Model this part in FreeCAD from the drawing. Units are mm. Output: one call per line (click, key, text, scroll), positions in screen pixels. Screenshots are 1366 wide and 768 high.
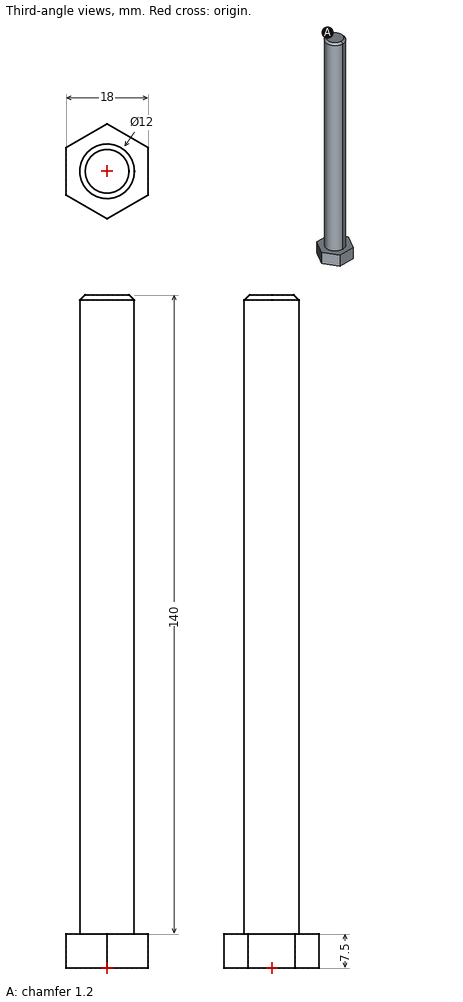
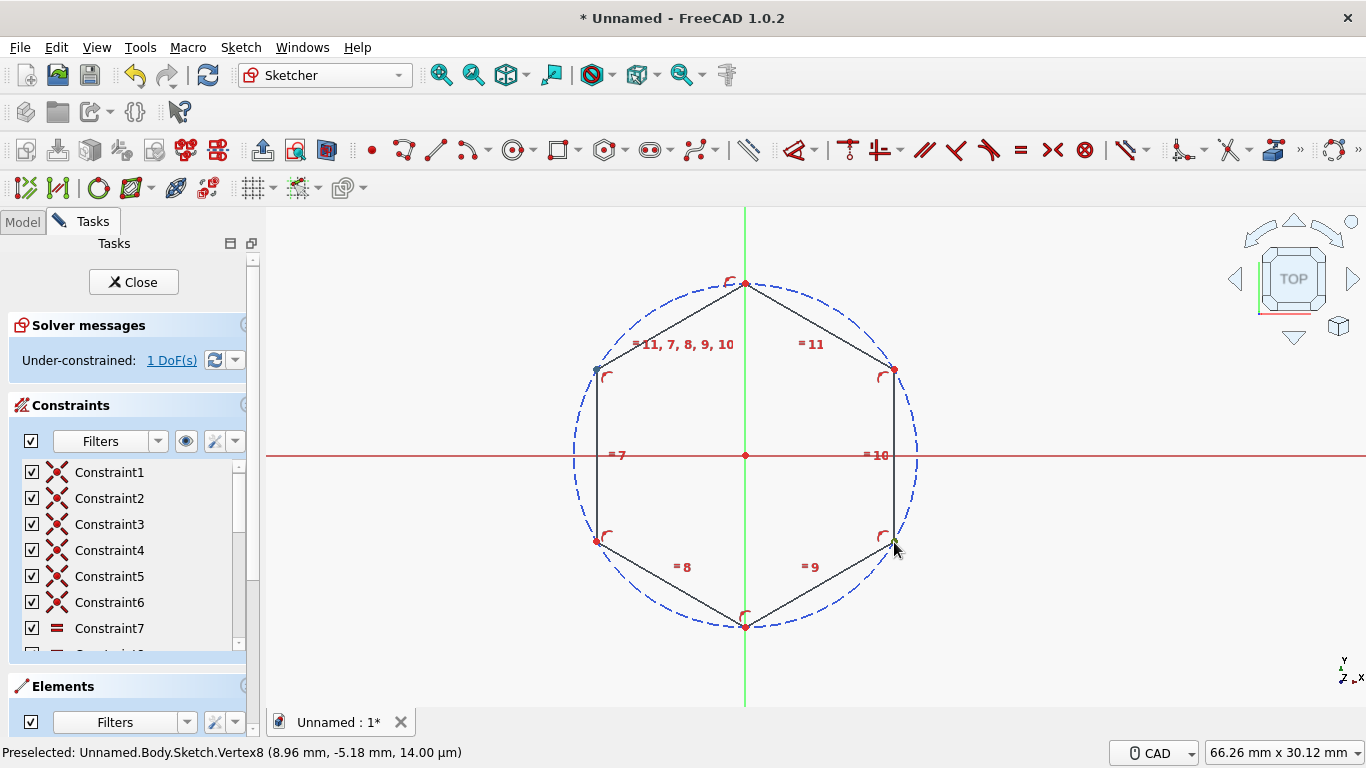
key(l)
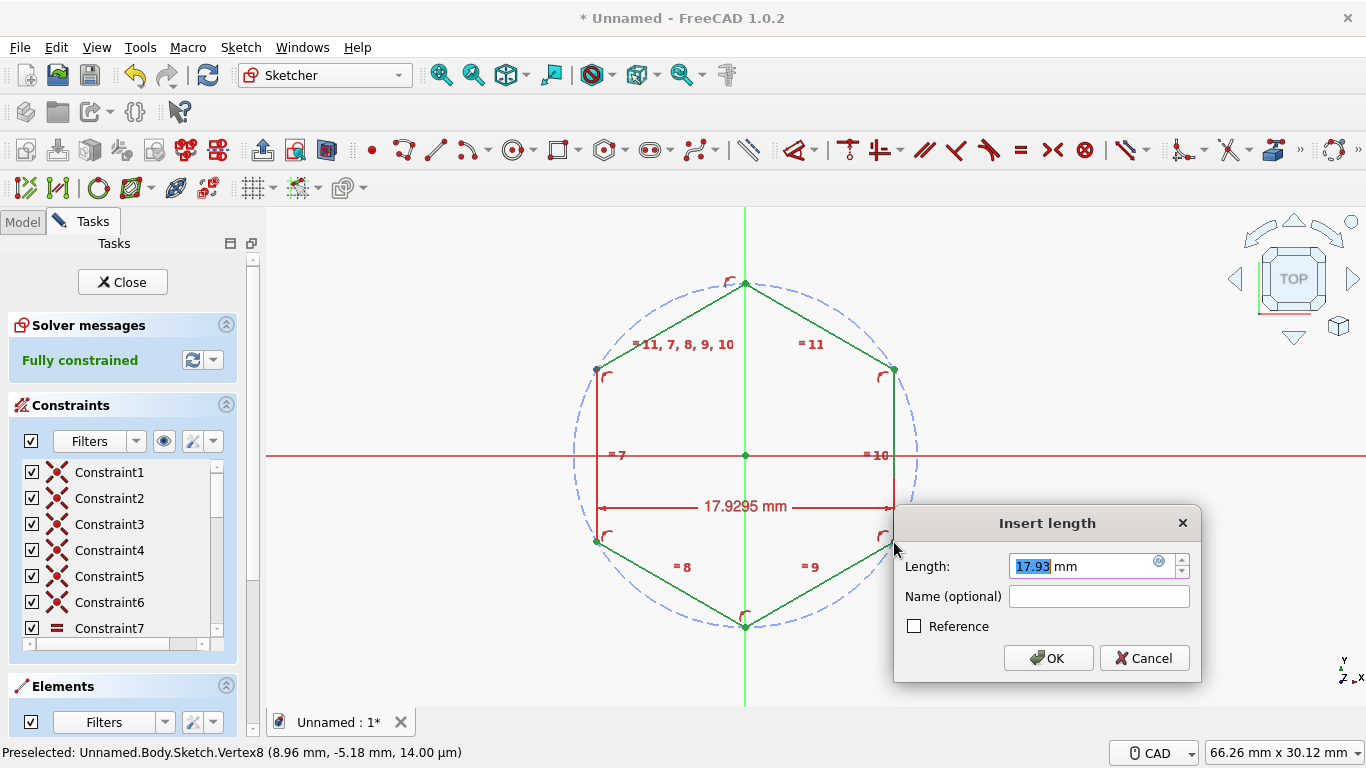
text(18)
key(Return)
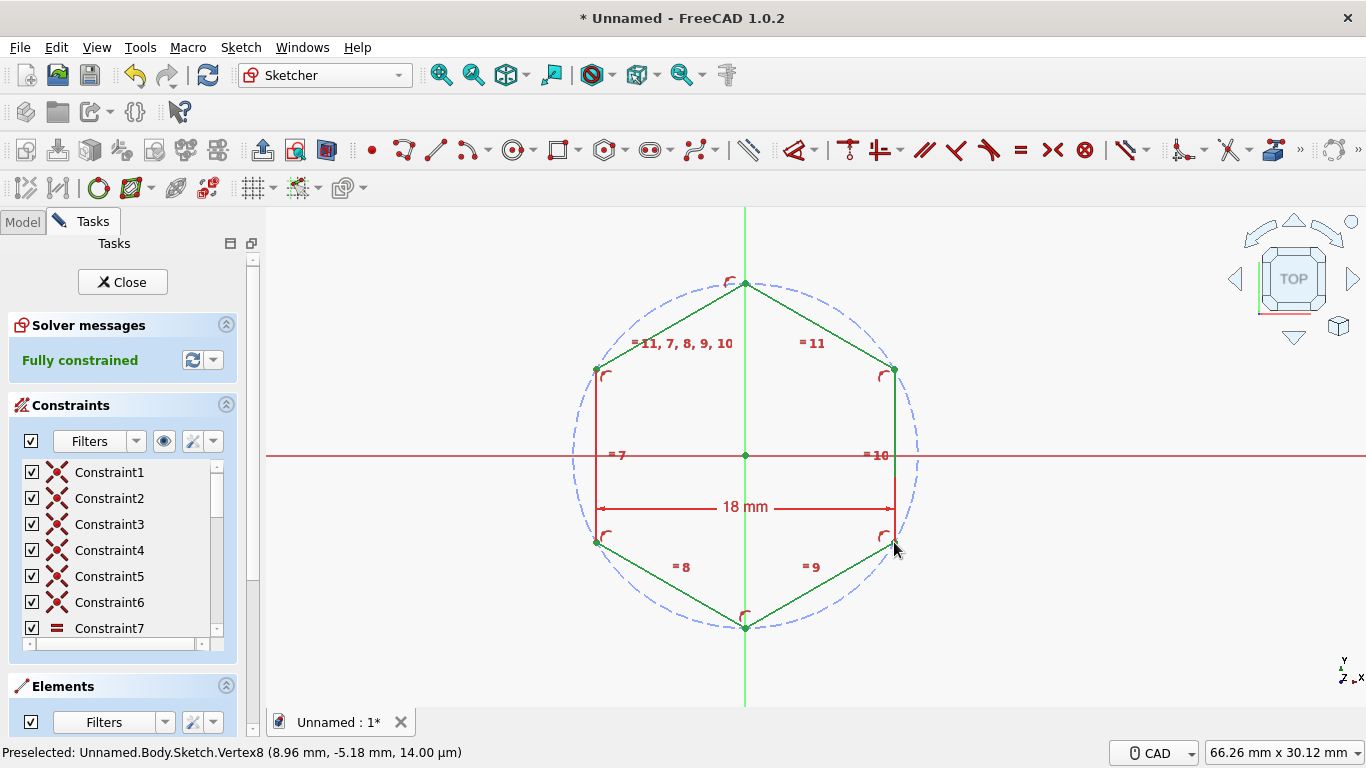
click(123, 282)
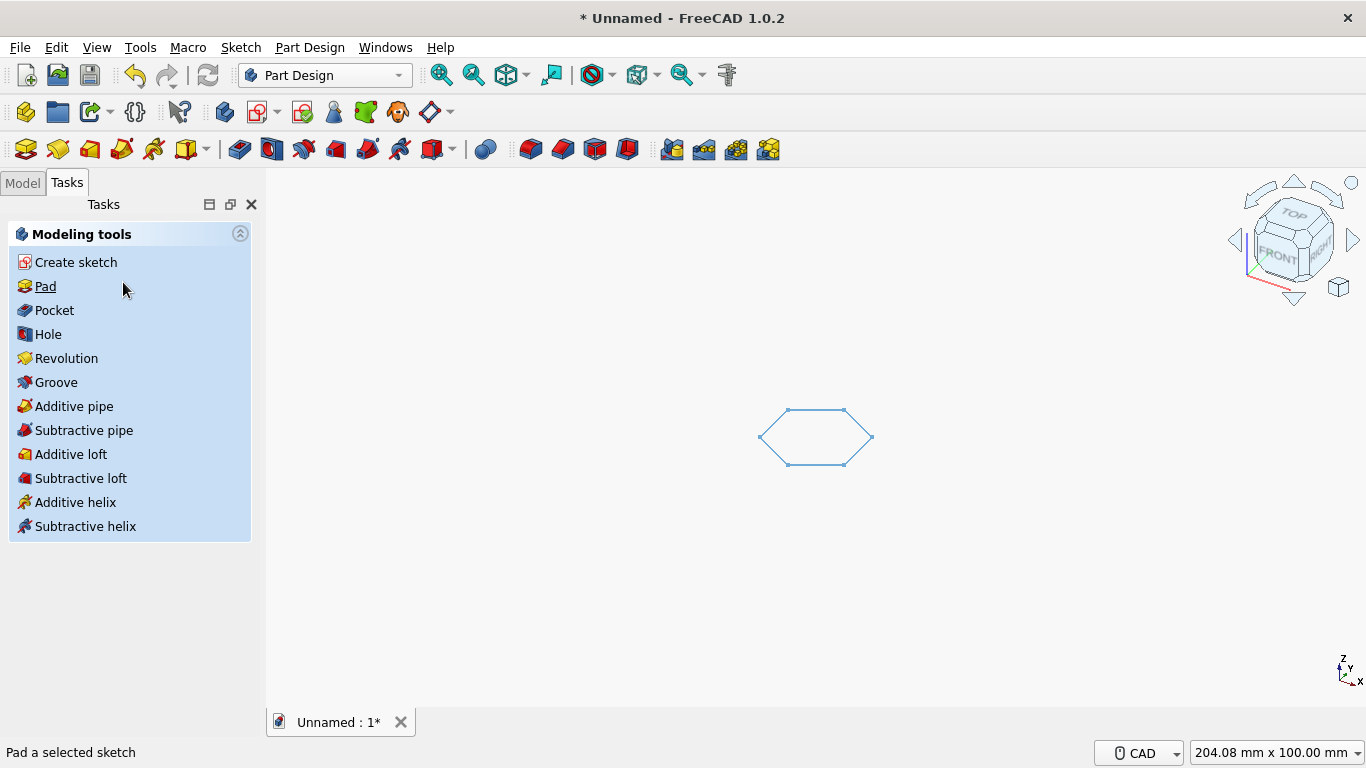
click(26, 150)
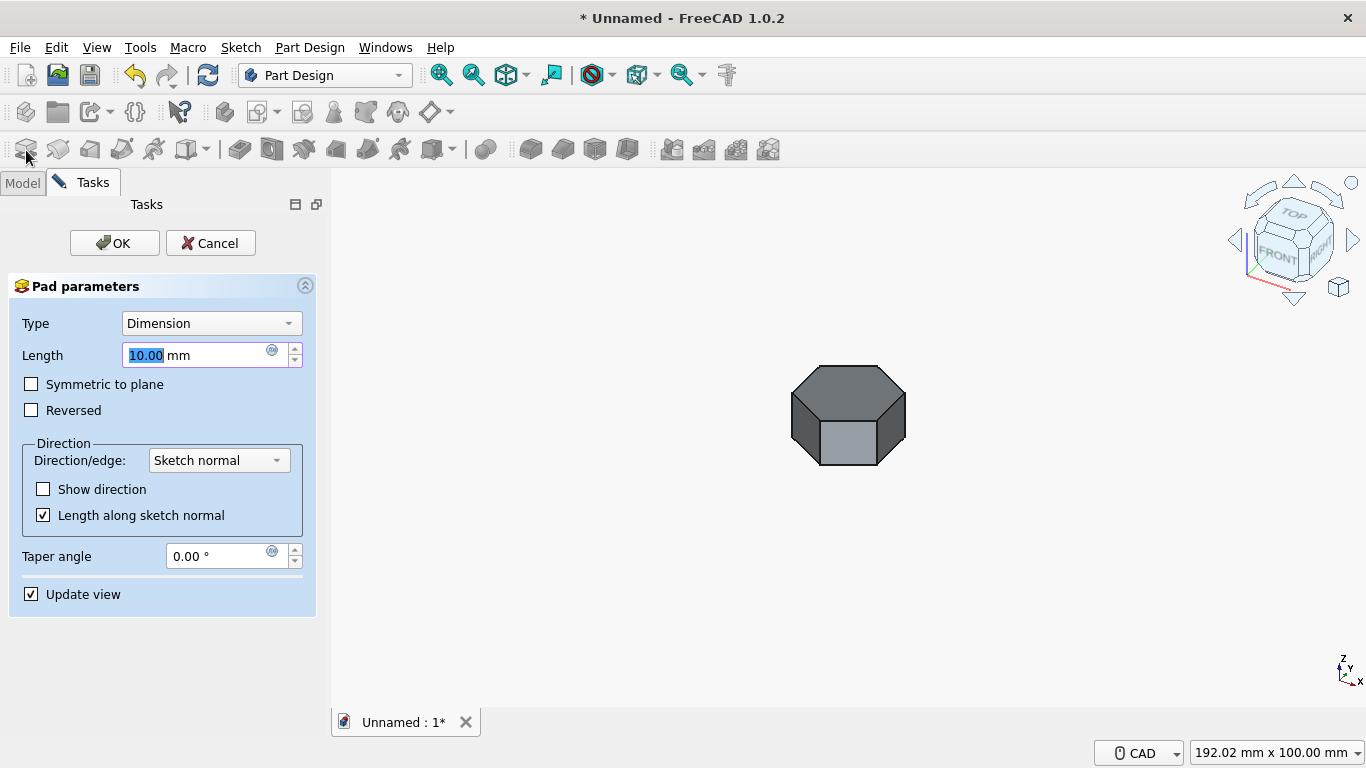
text(7.5)
key(Tab)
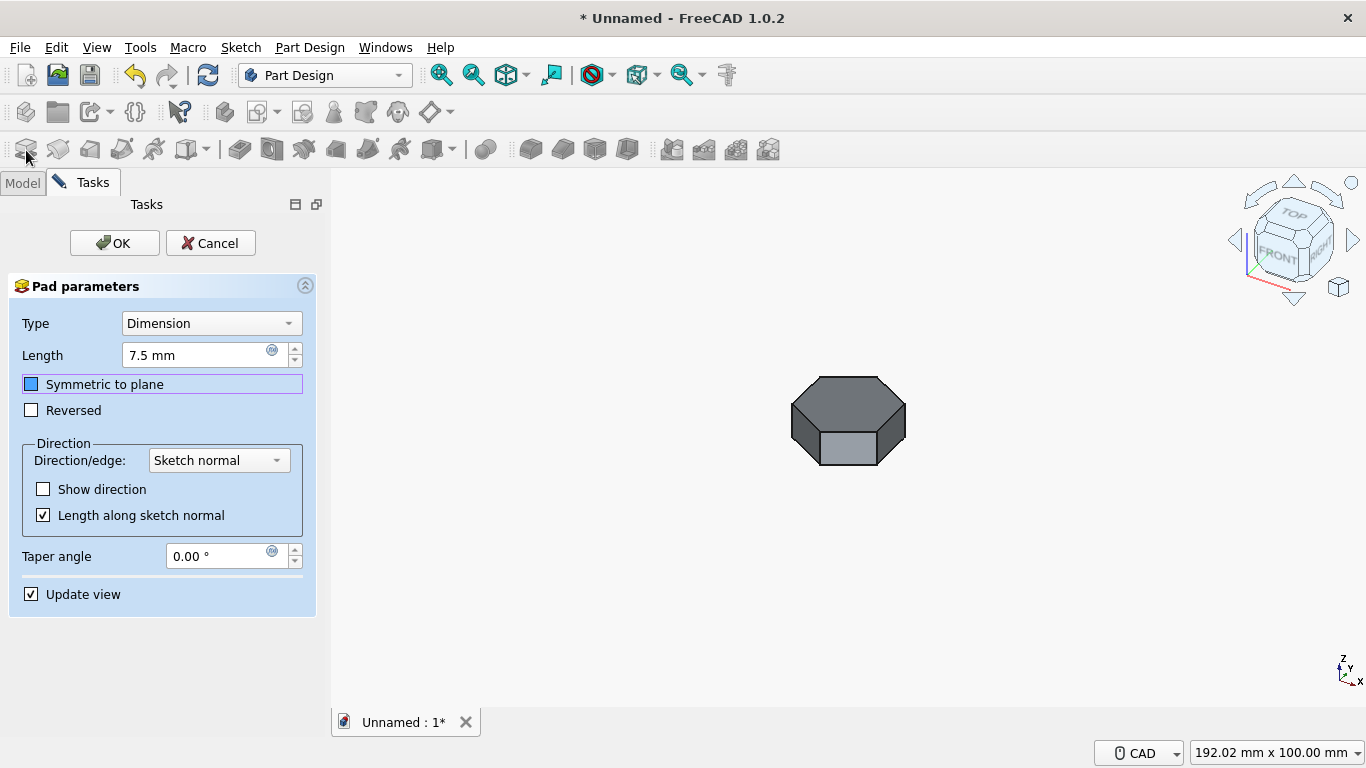
click(115, 243)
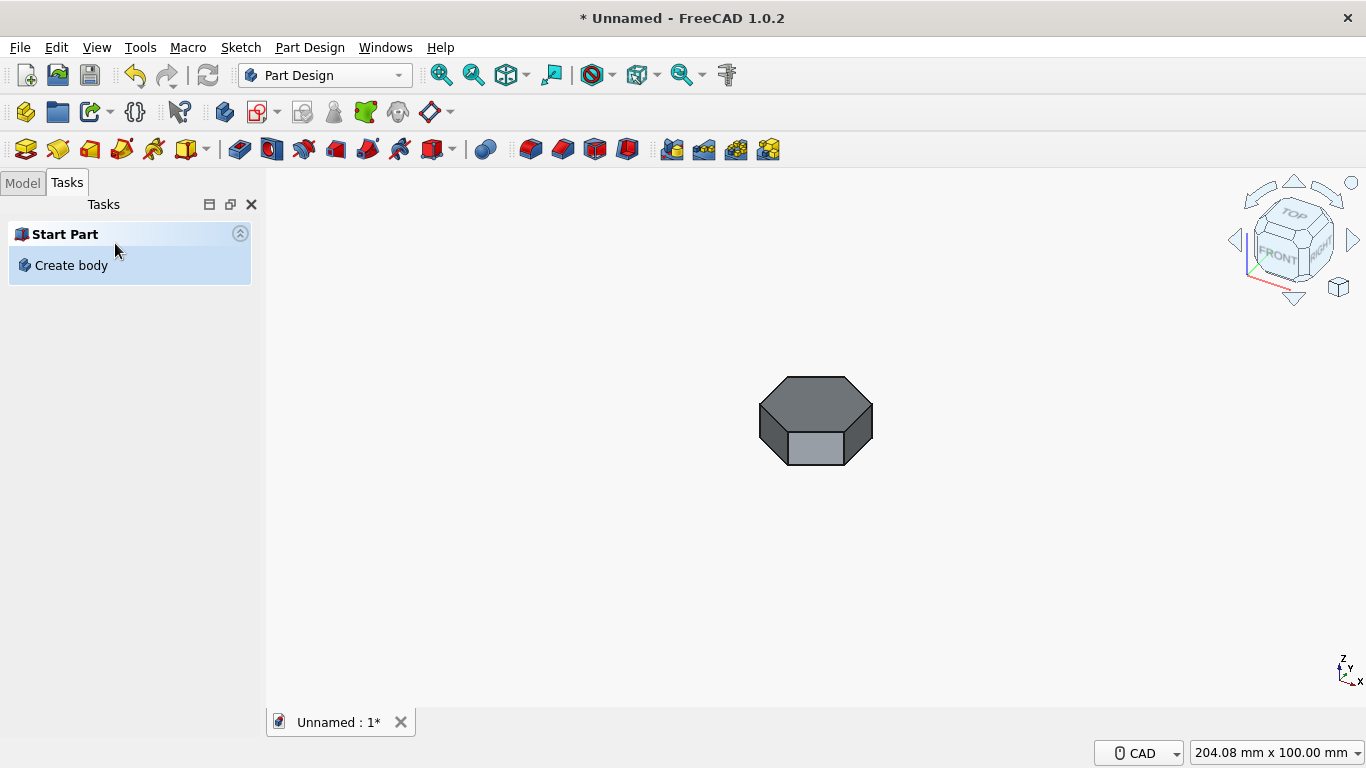
key(v)
key(f)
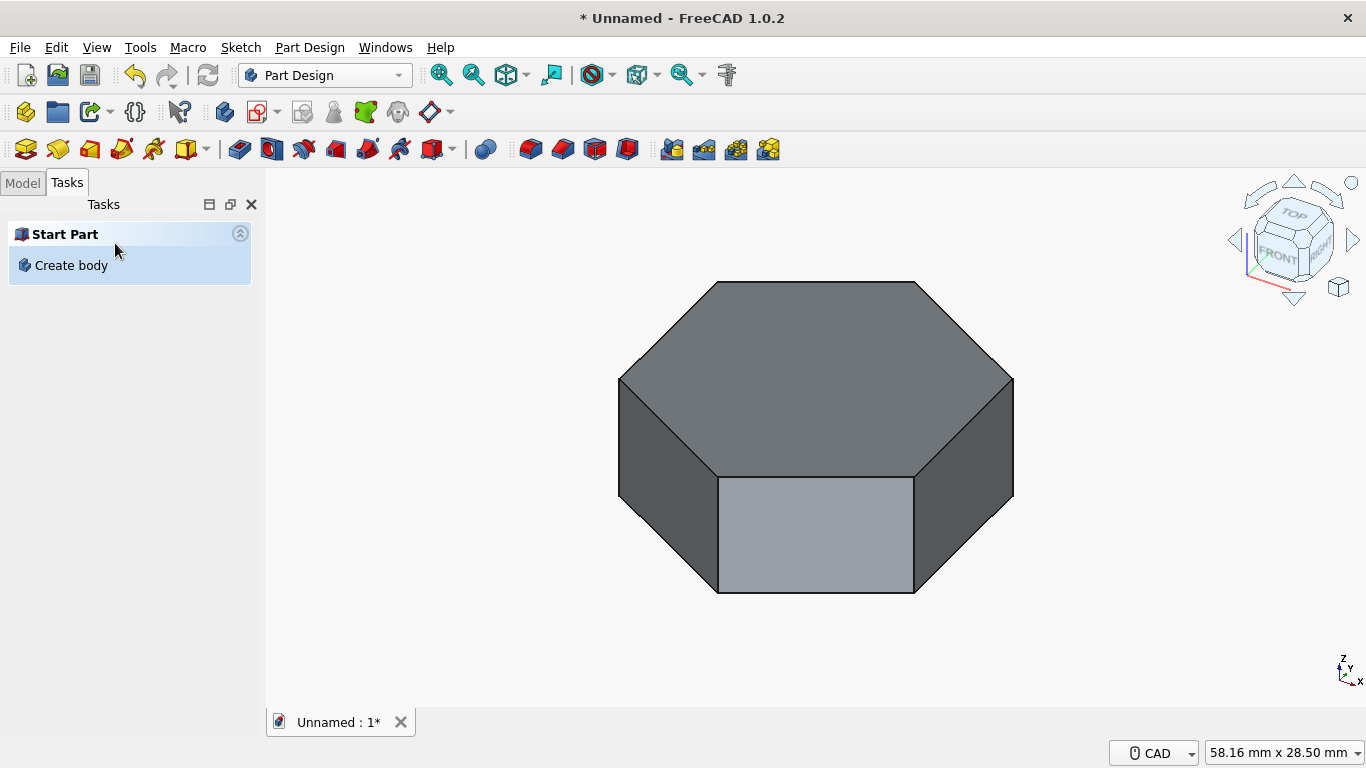
click(816, 378)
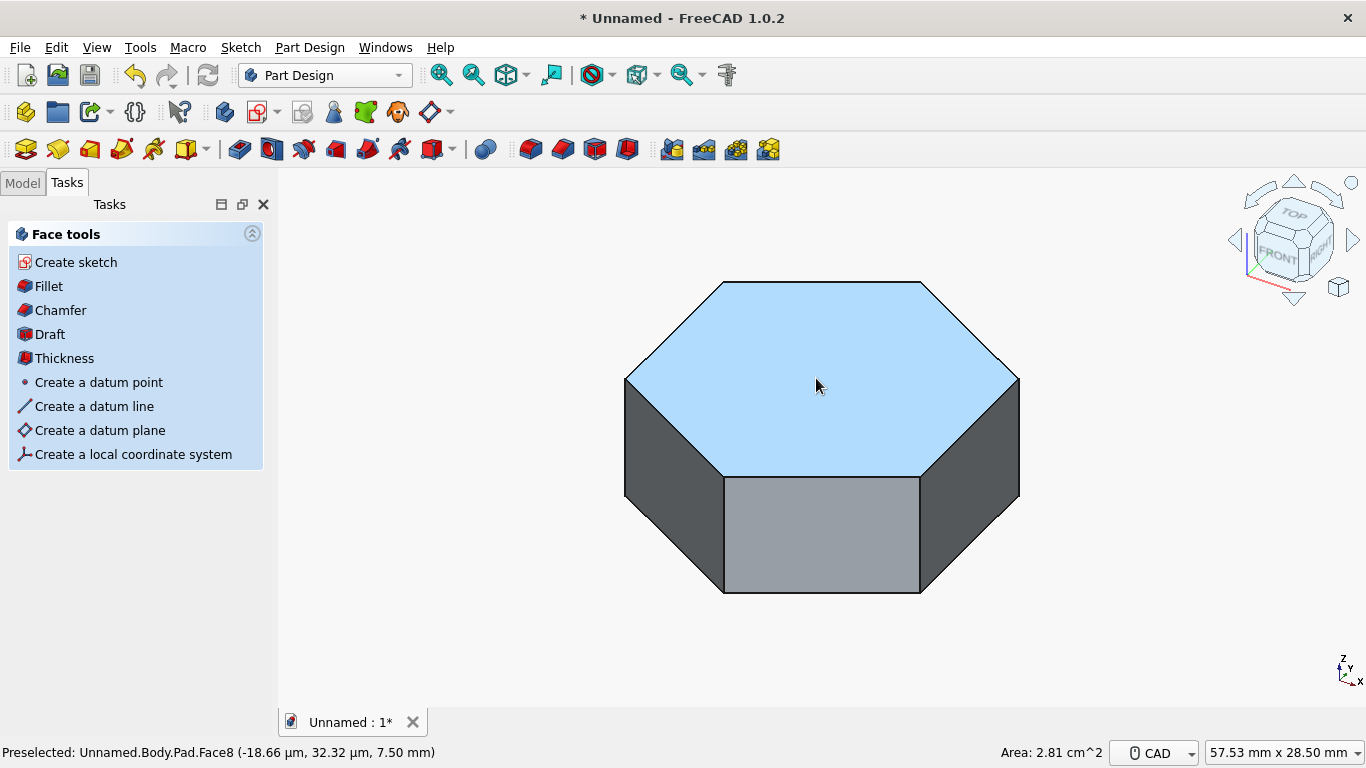
click(258, 112)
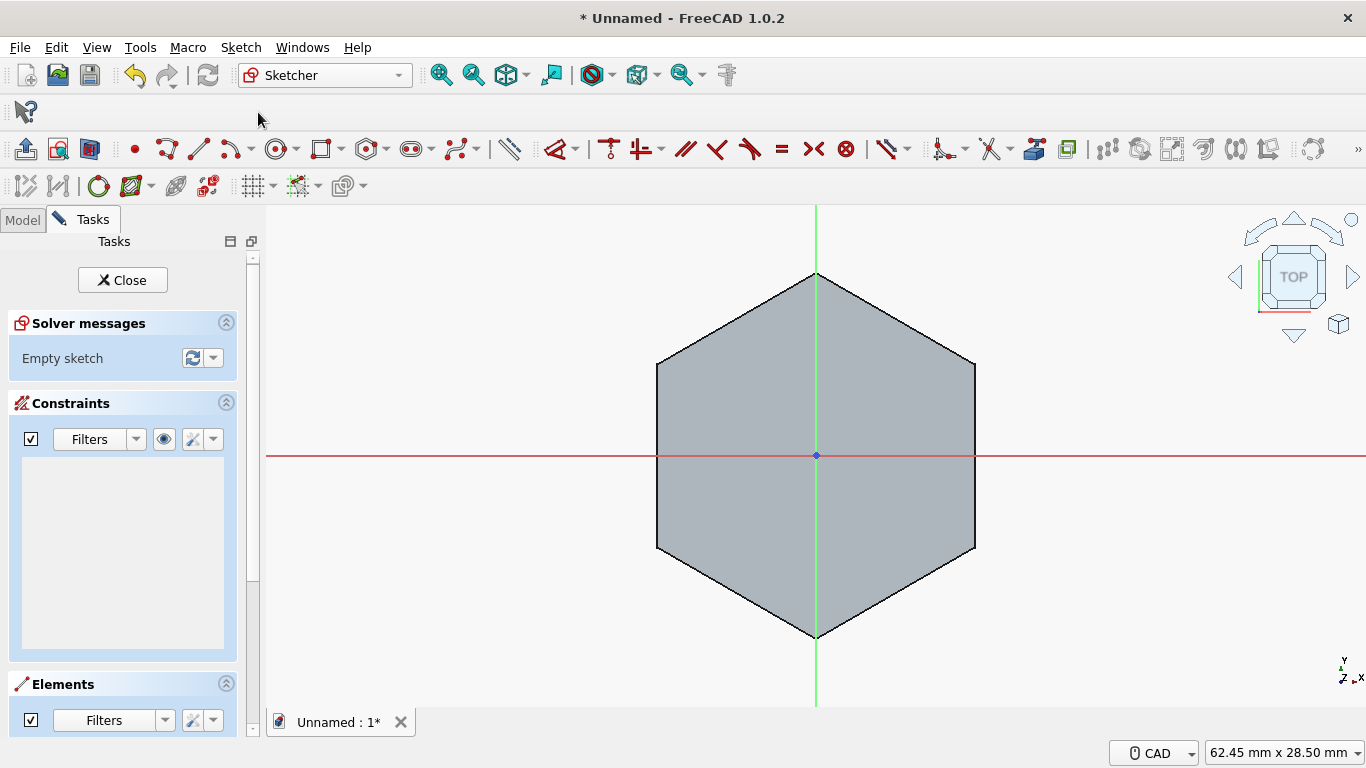
scroll(955, 456, up, 2)